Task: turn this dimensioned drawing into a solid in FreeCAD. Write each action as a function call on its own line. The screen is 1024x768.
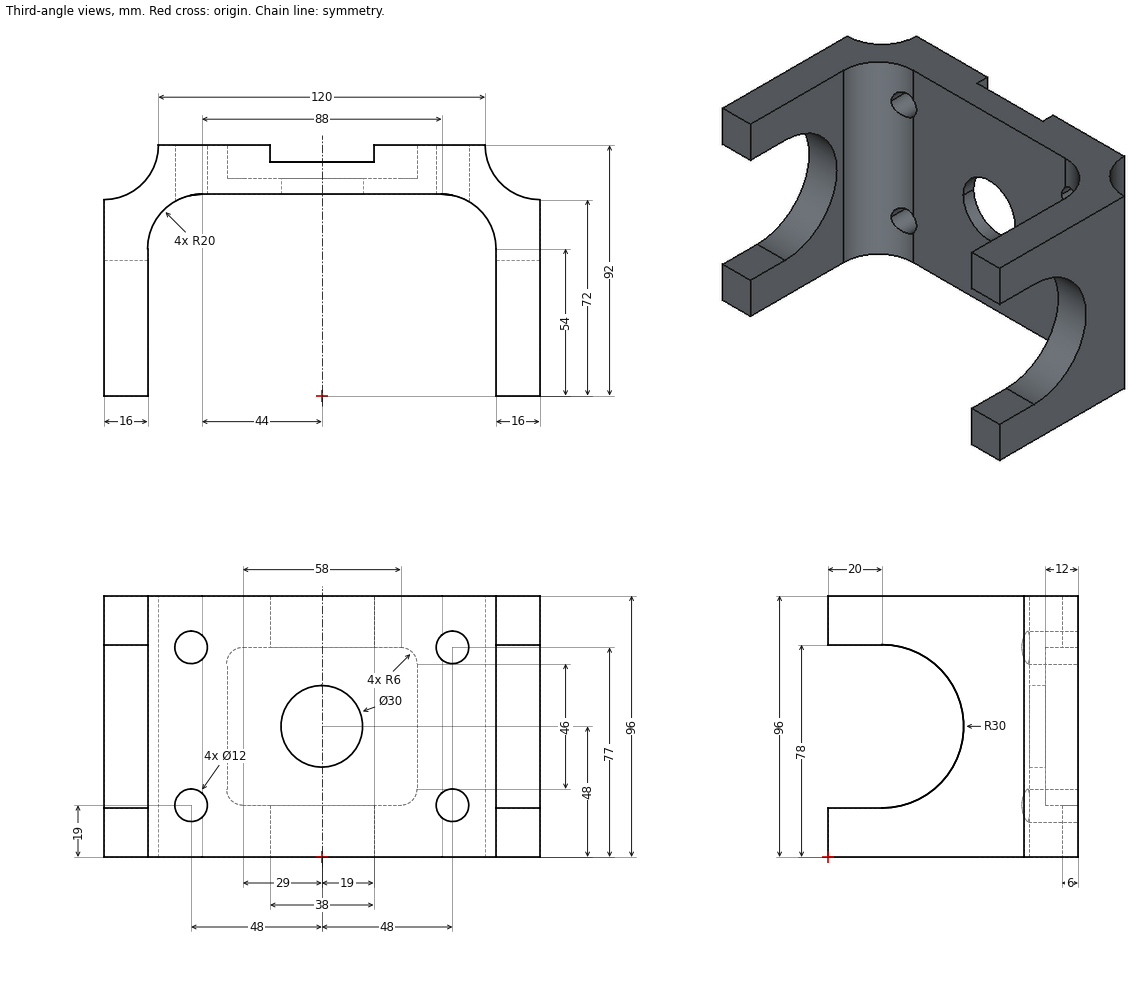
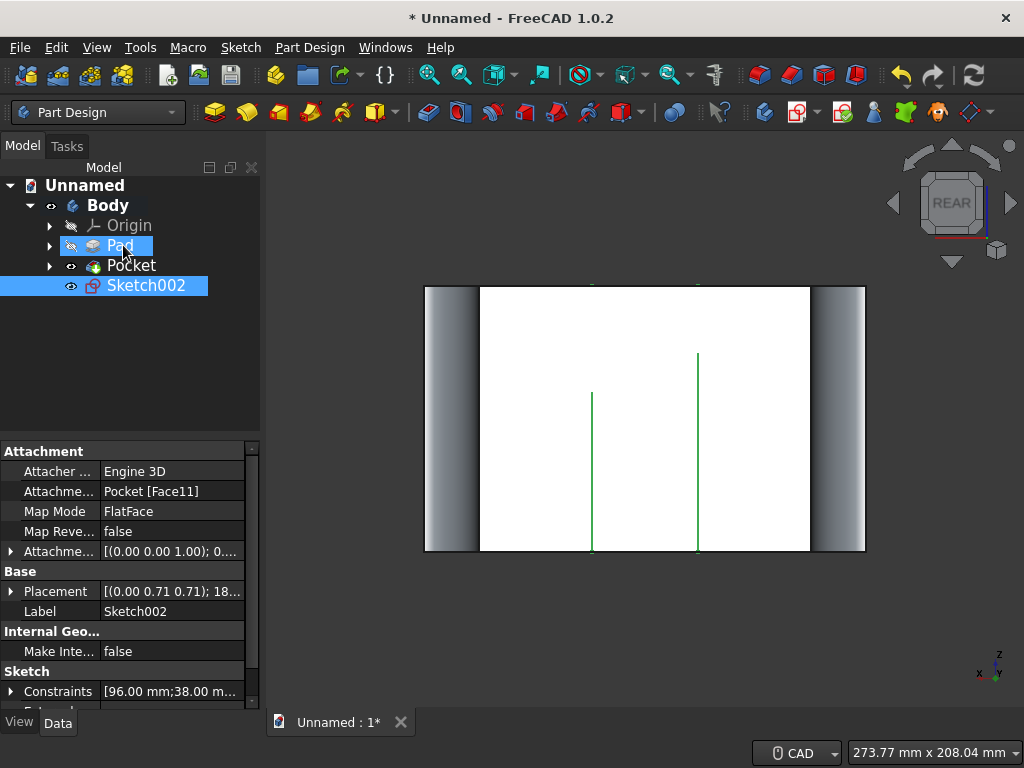
click(430, 112)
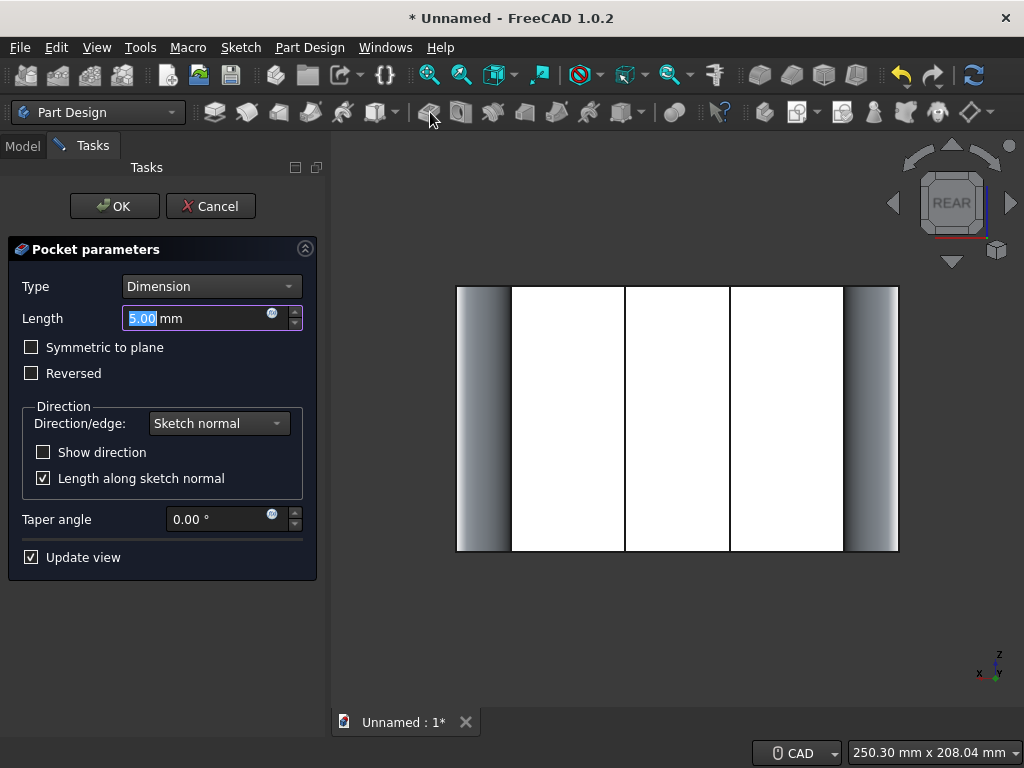
text(6)
key(Tab)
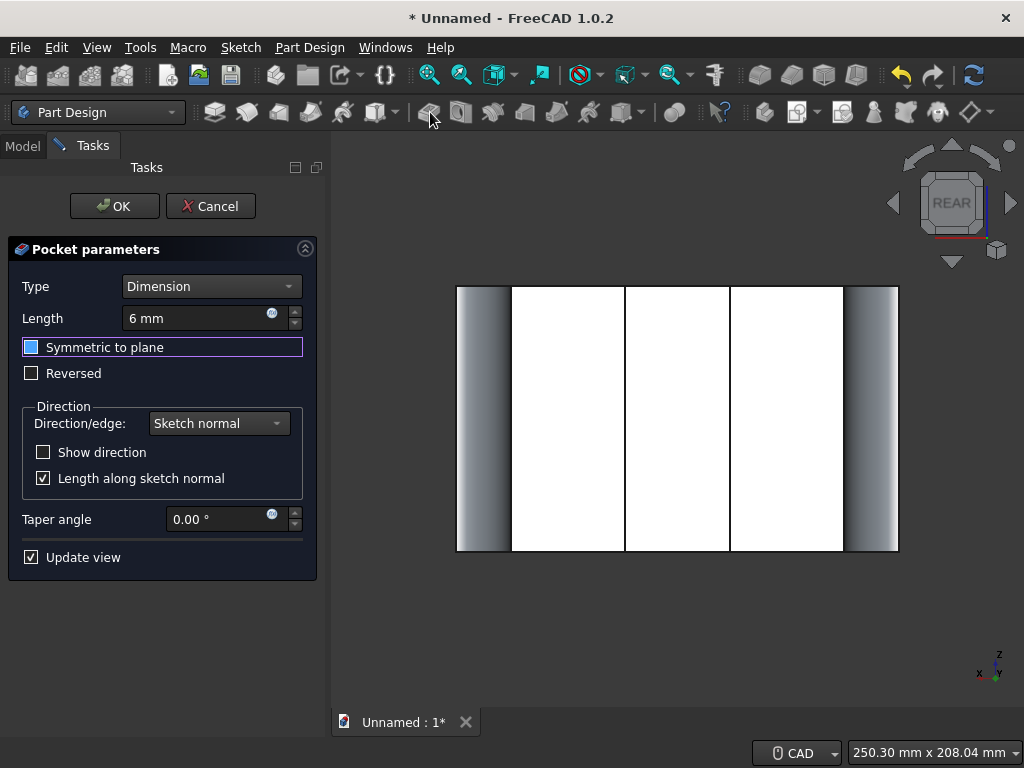
click(115, 206)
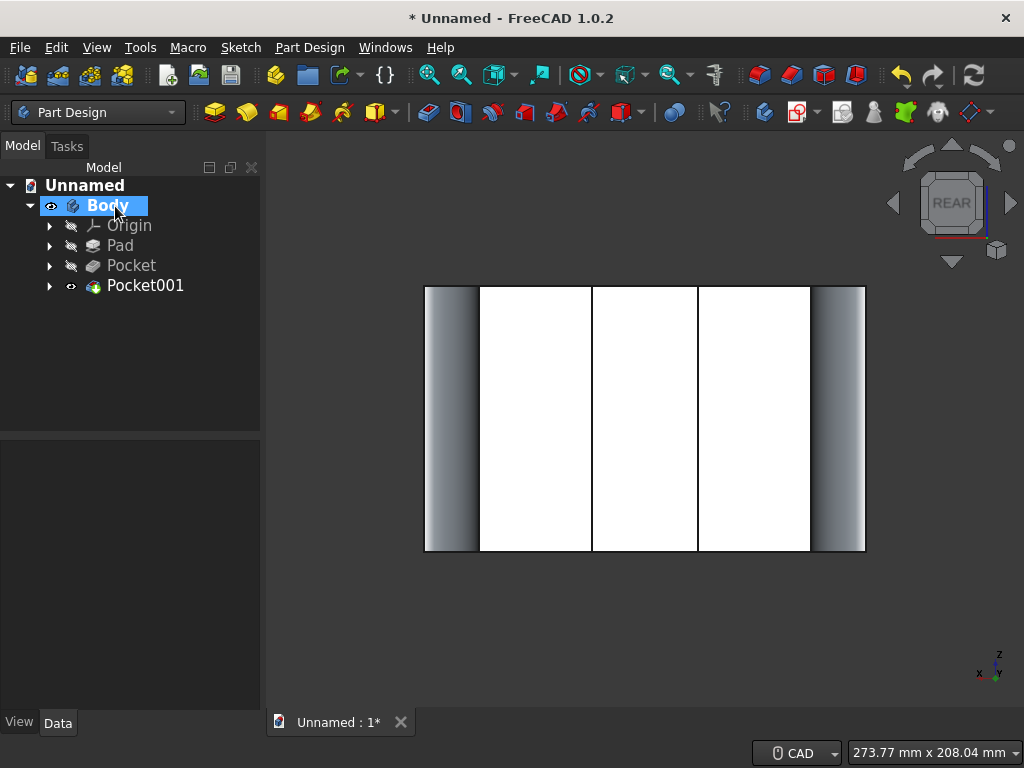
click(645, 342)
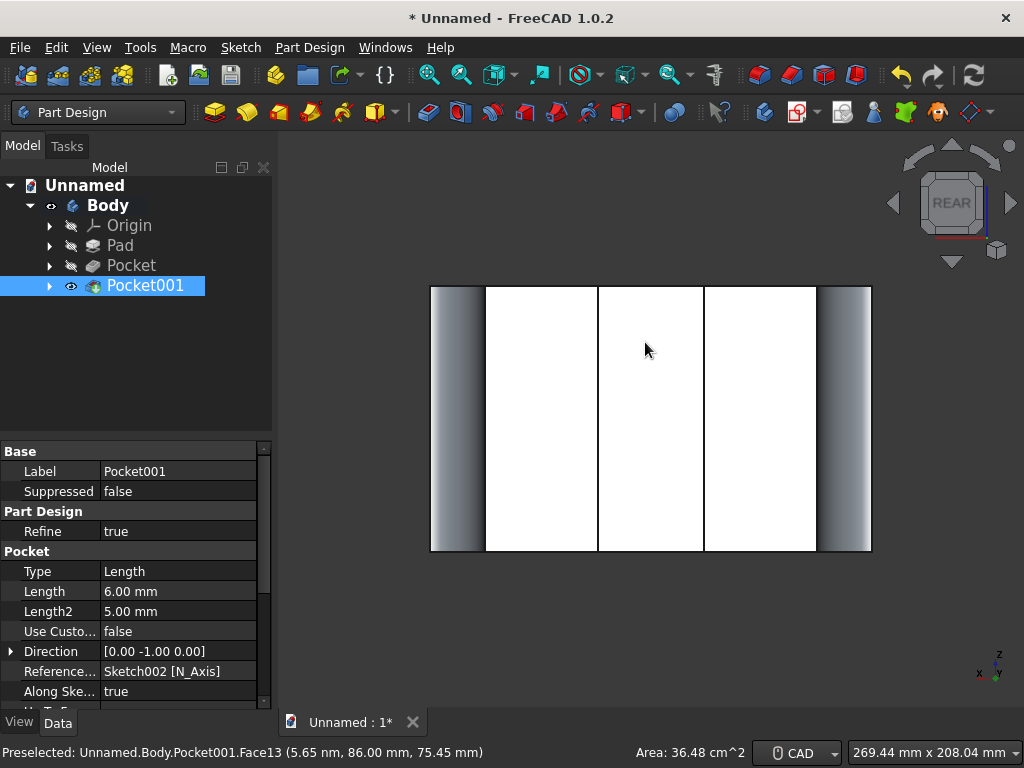
click(798, 112)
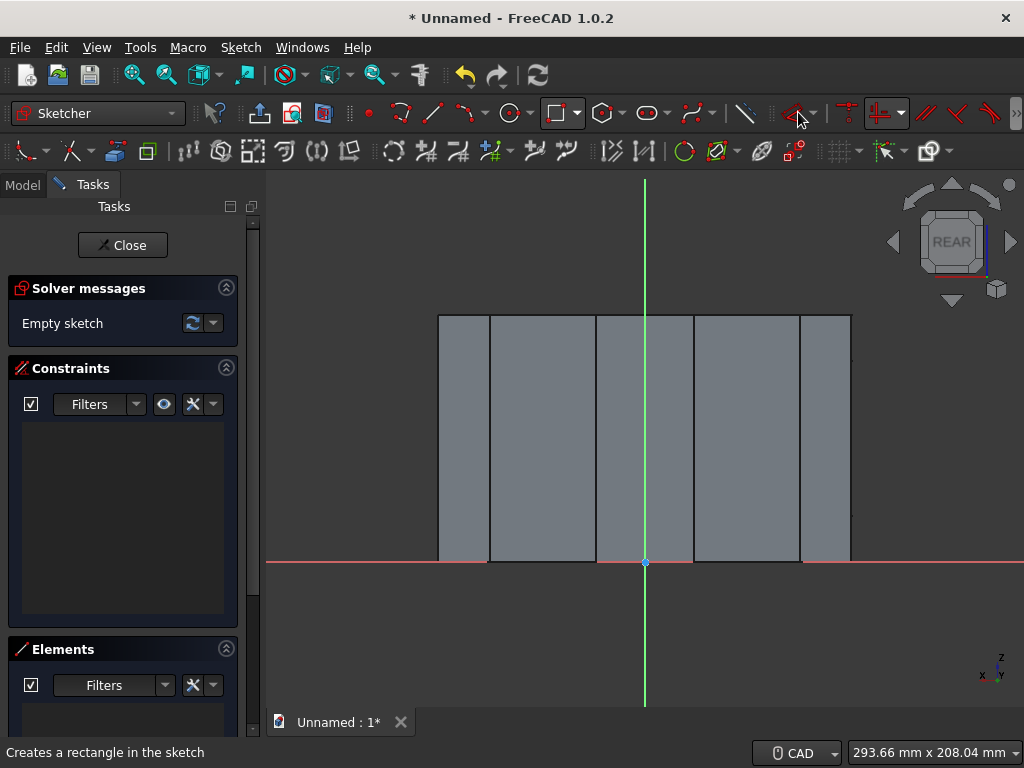
click(324, 114)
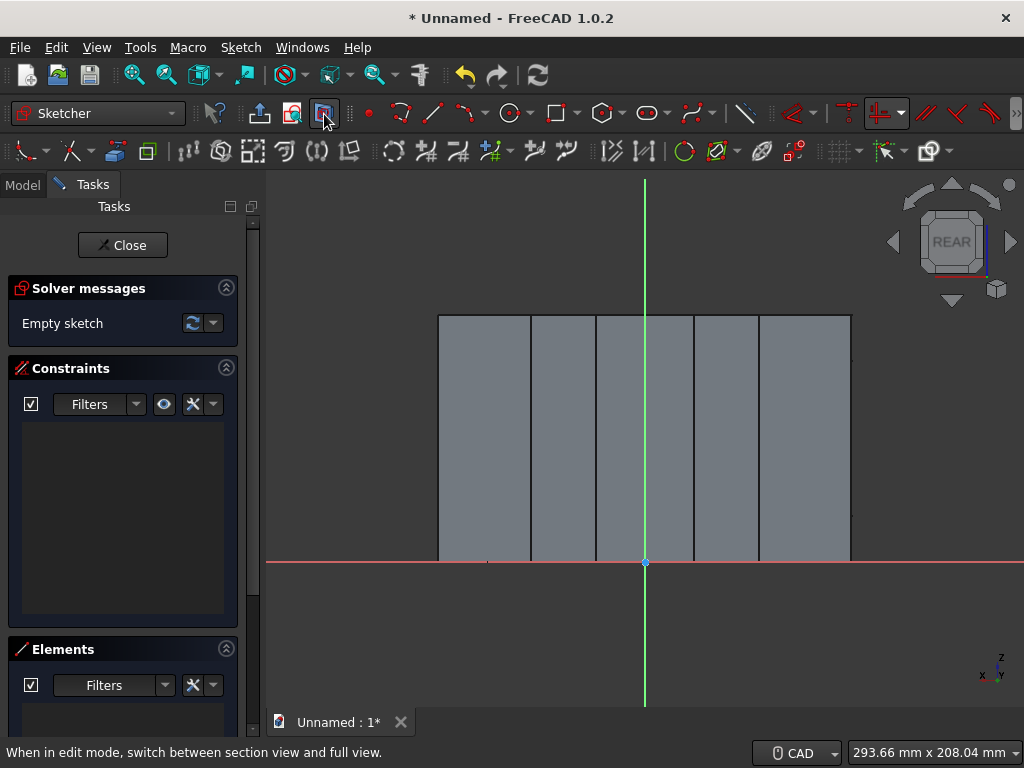
scroll(701, 516, up, 4)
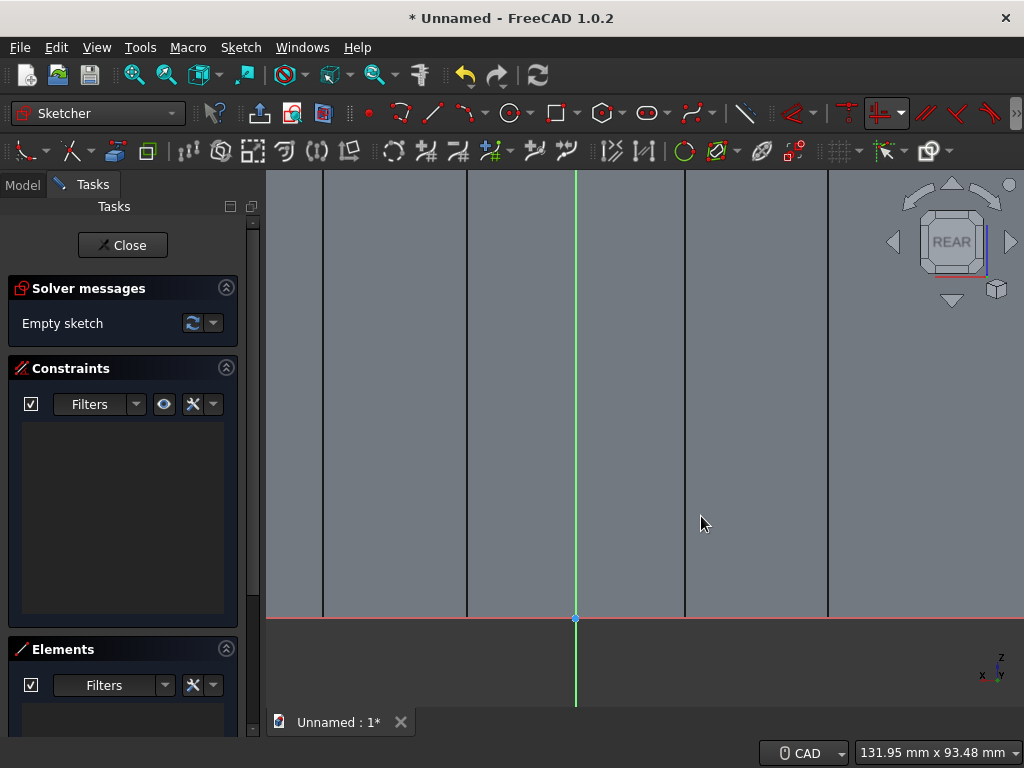
click(510, 114)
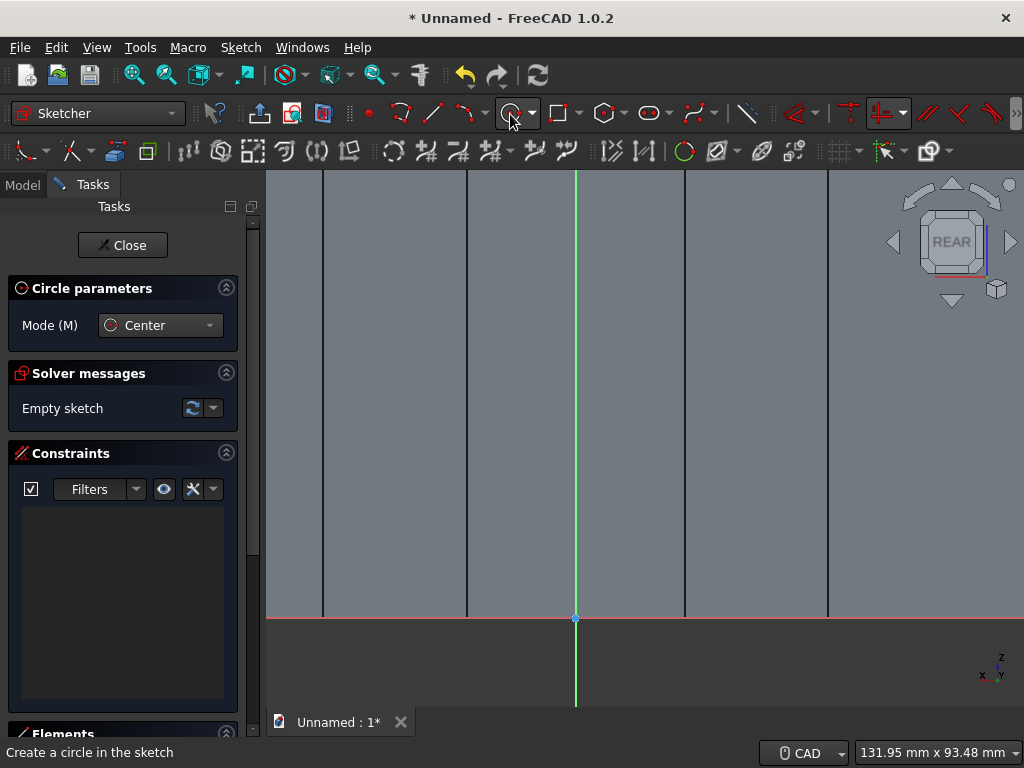
click(576, 343)
move(637, 282)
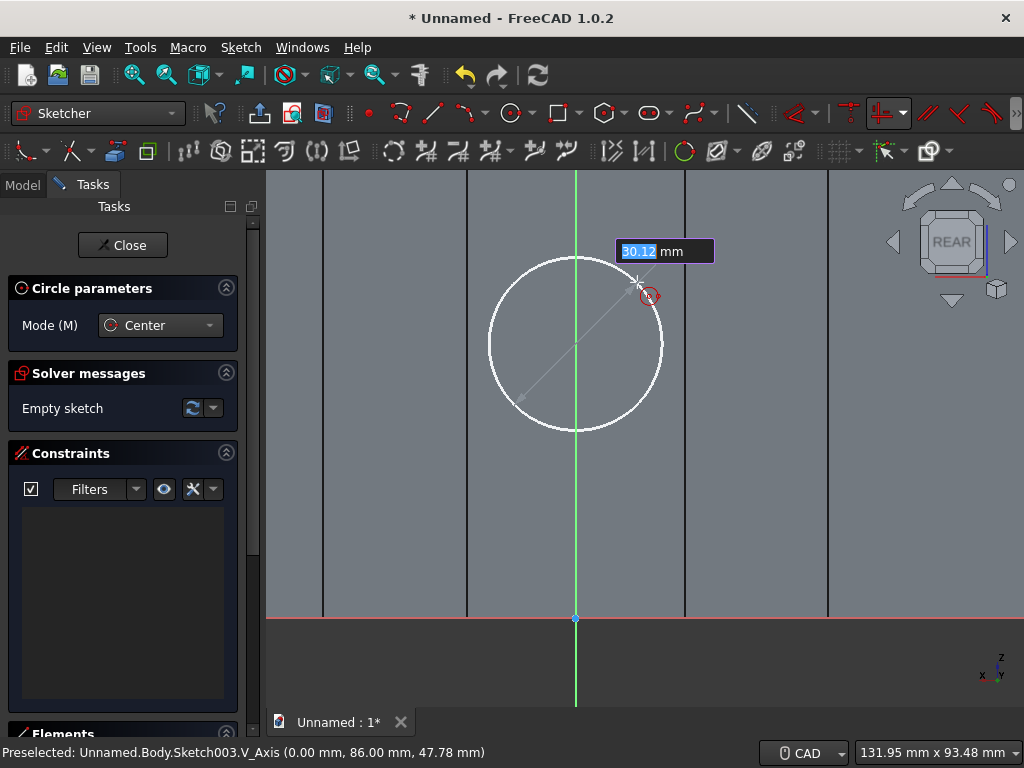
text(30)
key(Return)
key(Escape)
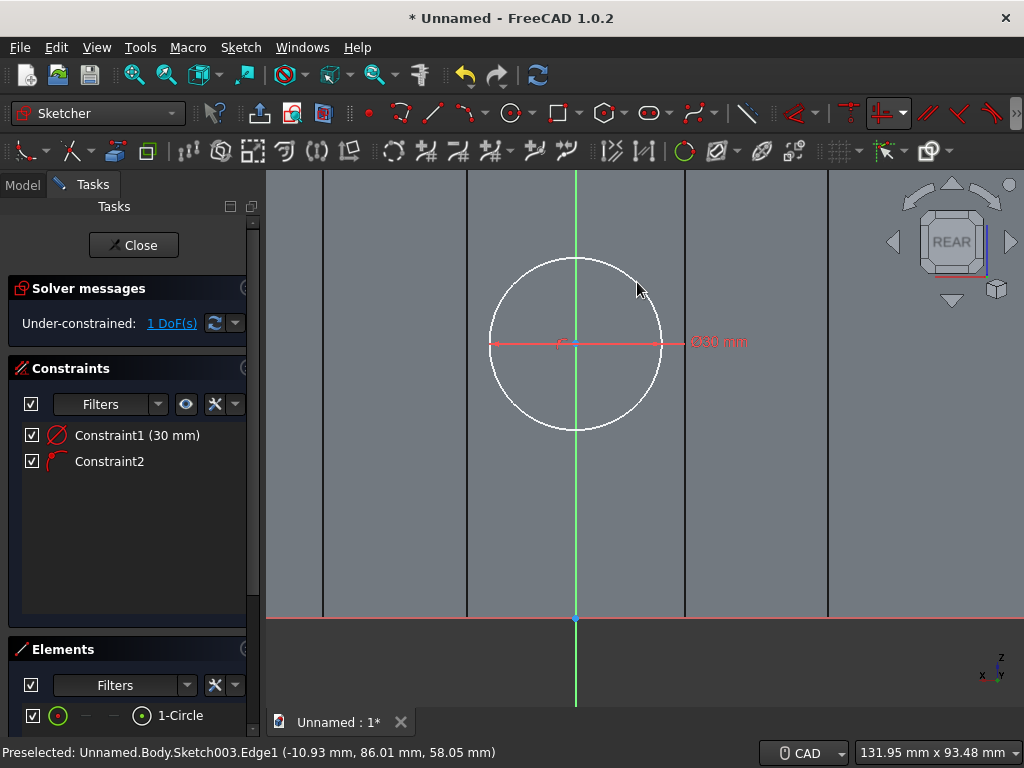
click(794, 114)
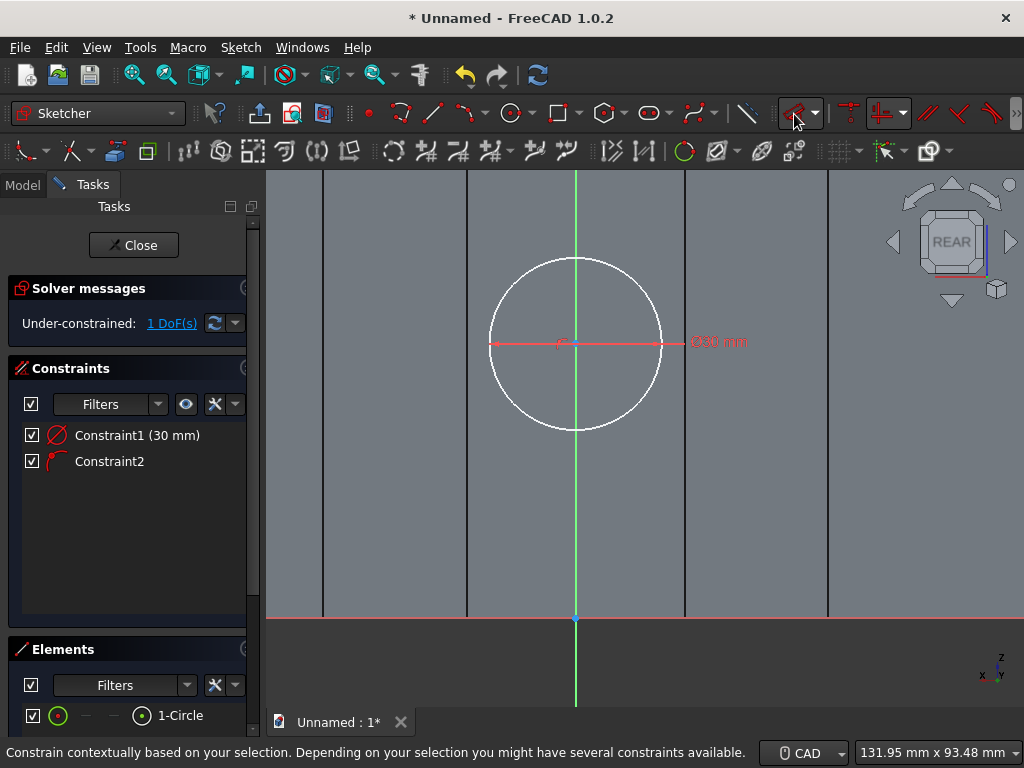
click(576, 344)
click(610, 481)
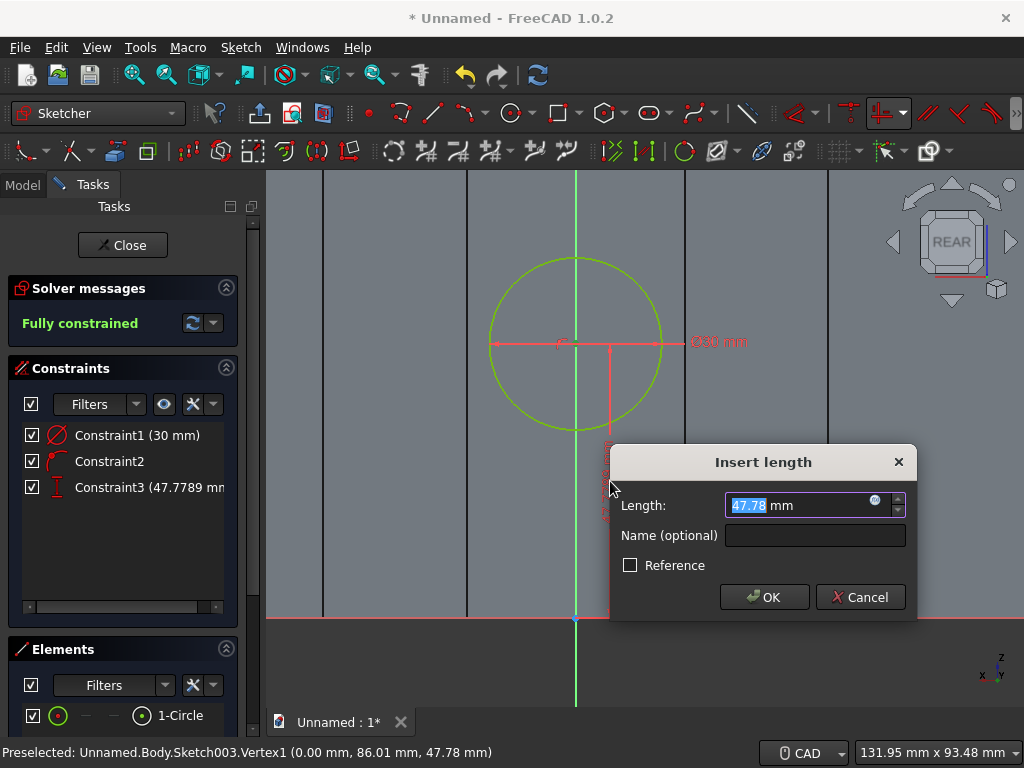
text(48)
key(Return)
key(Escape)